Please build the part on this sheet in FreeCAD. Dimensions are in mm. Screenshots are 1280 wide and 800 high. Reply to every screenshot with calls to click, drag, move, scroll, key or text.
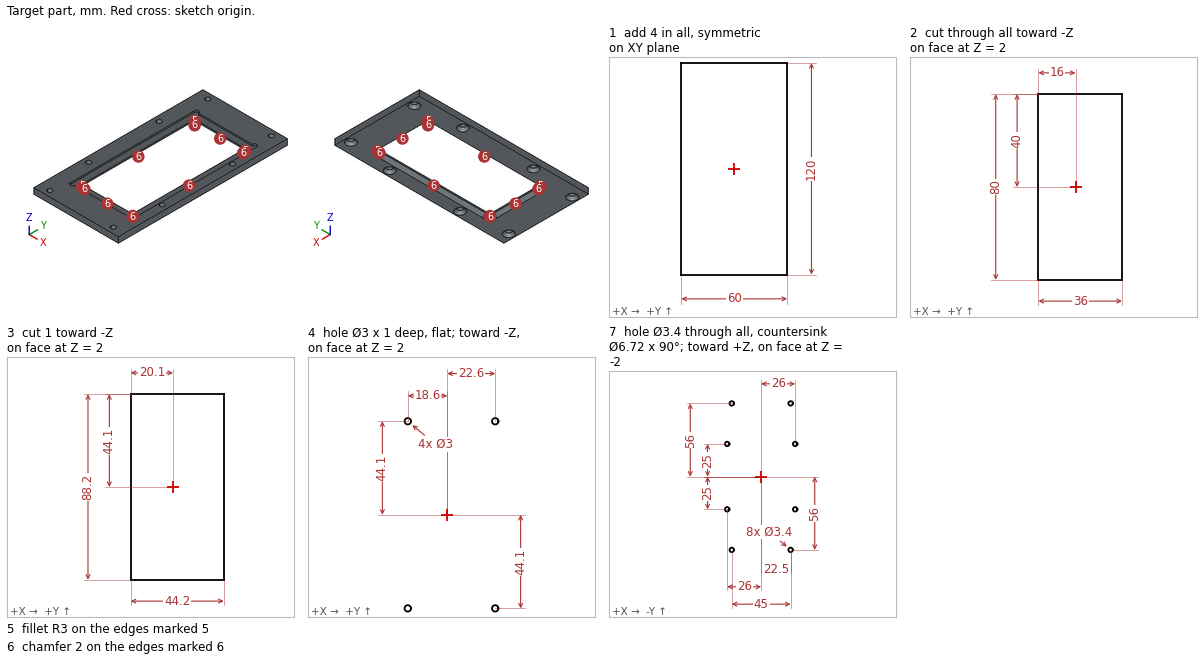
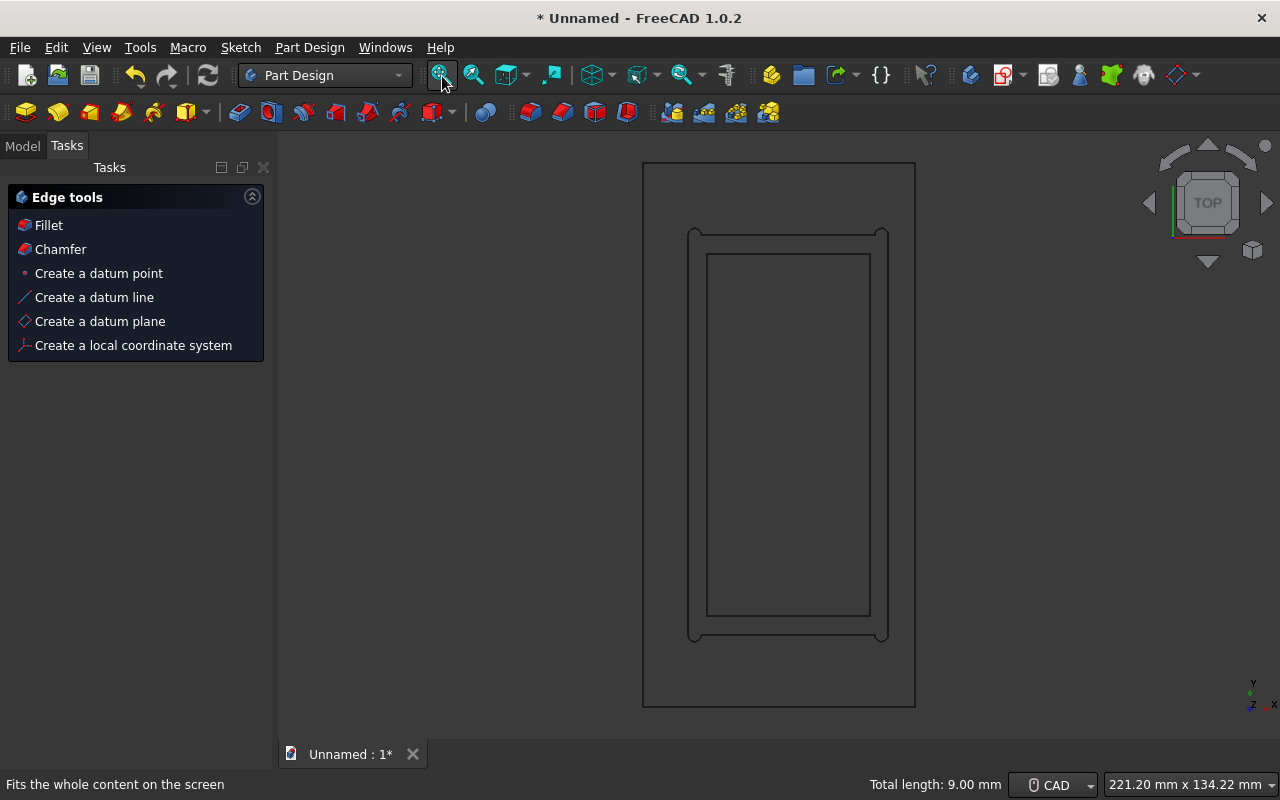
scroll(870, 253, up, 6)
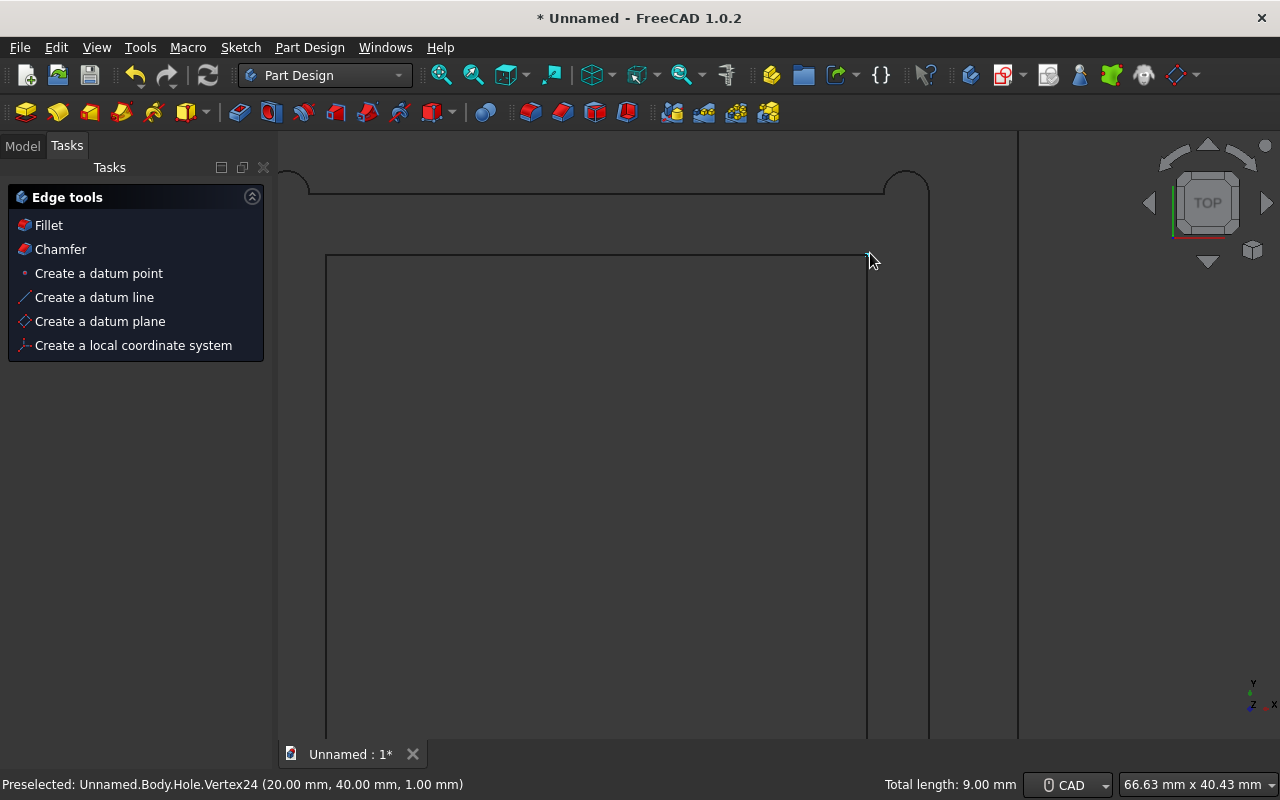
click(442, 76)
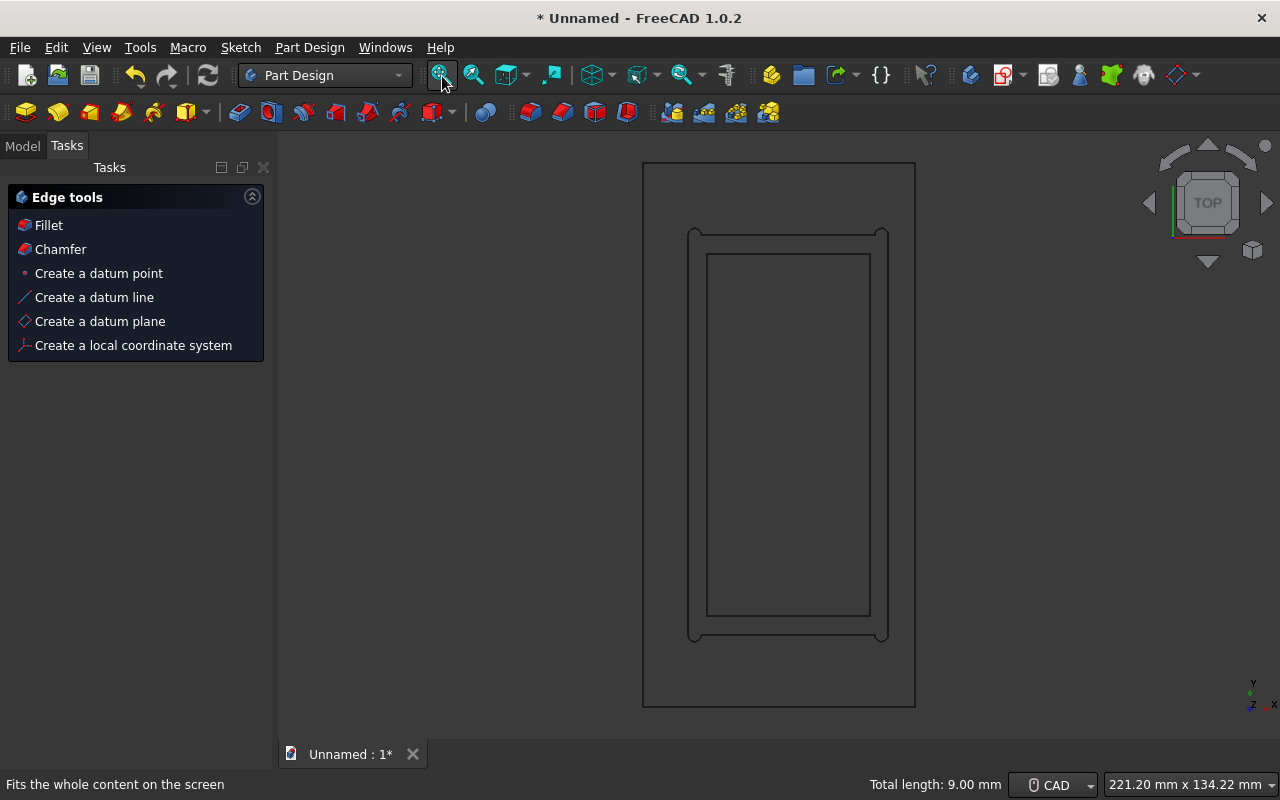
key(1)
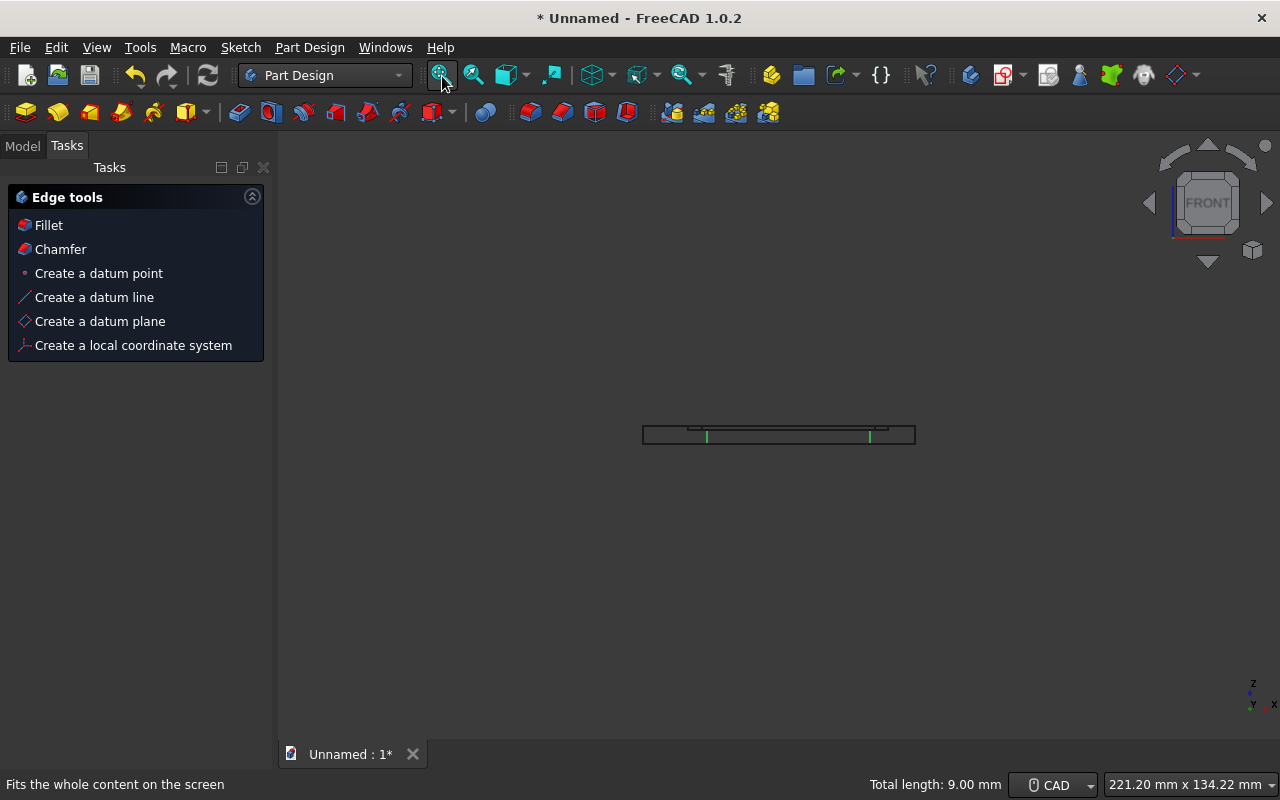
click(442, 76)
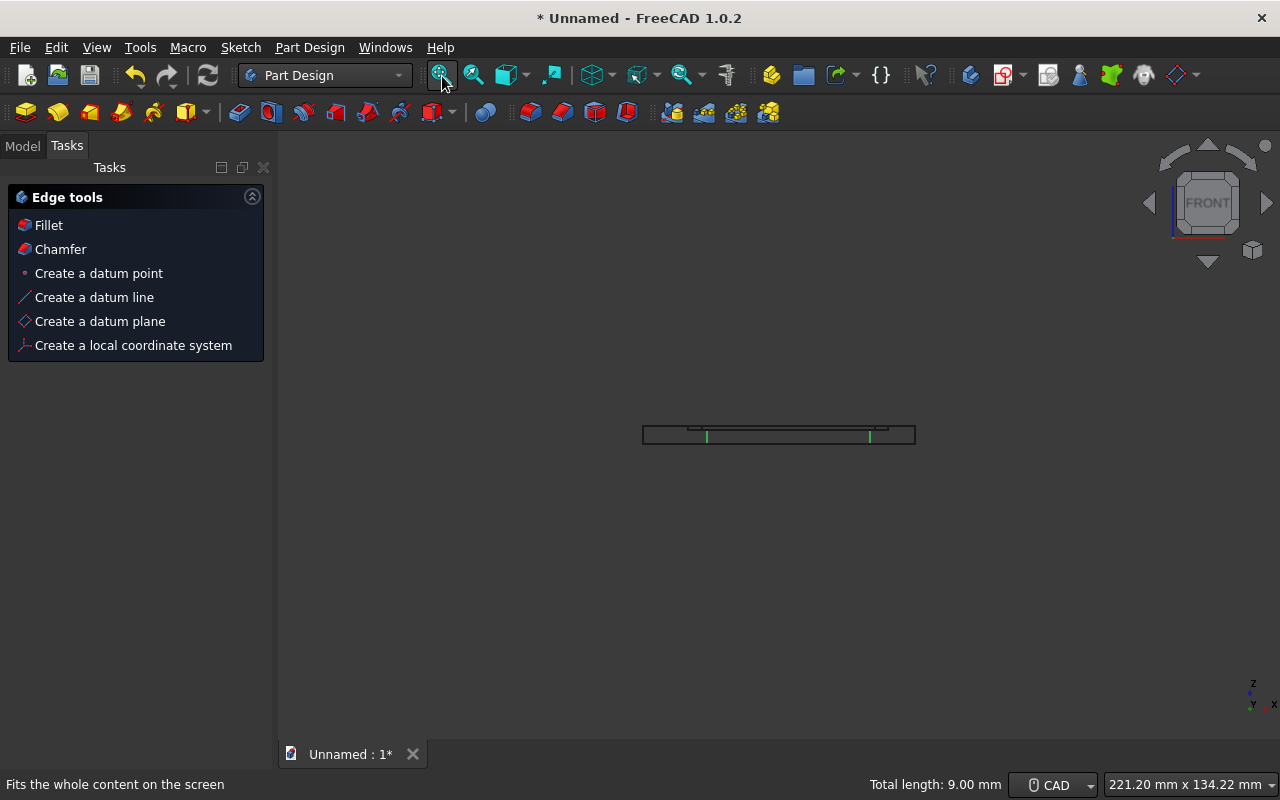
scroll(870, 436, up, 6)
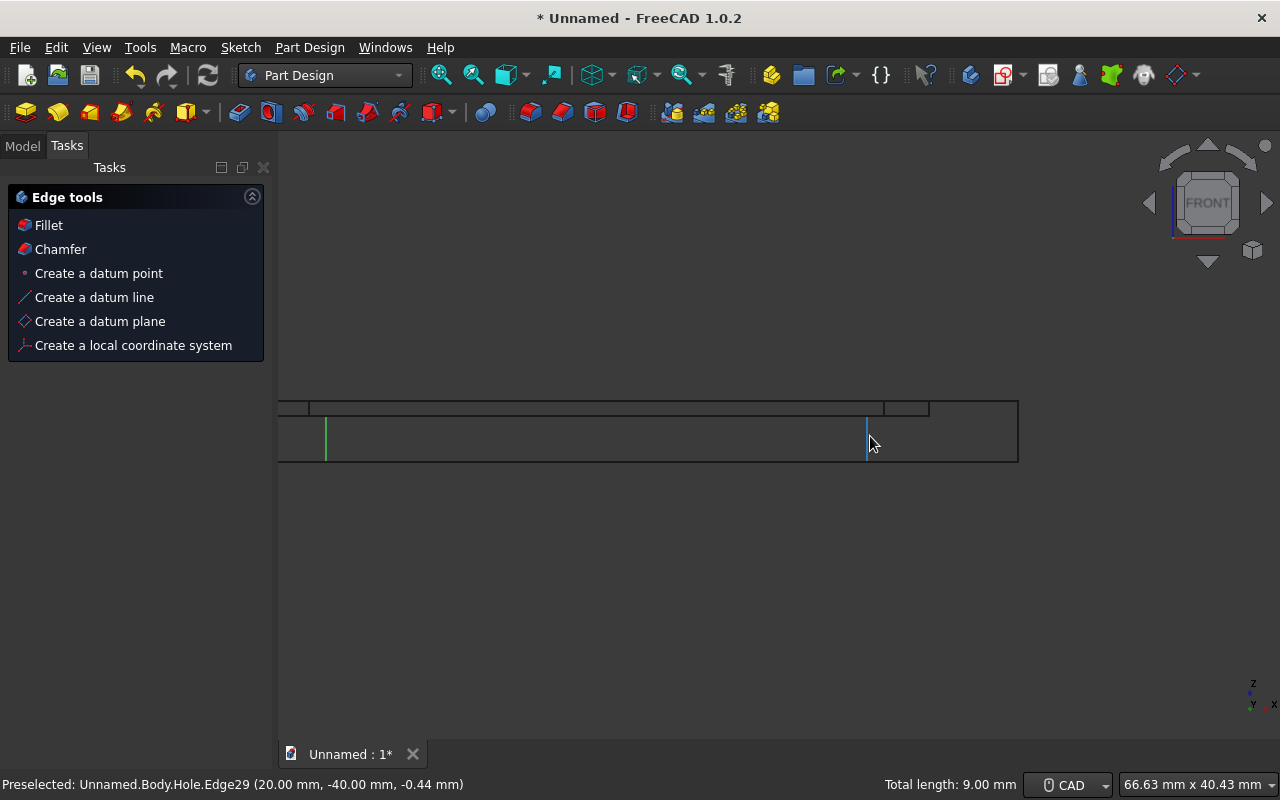
click(442, 76)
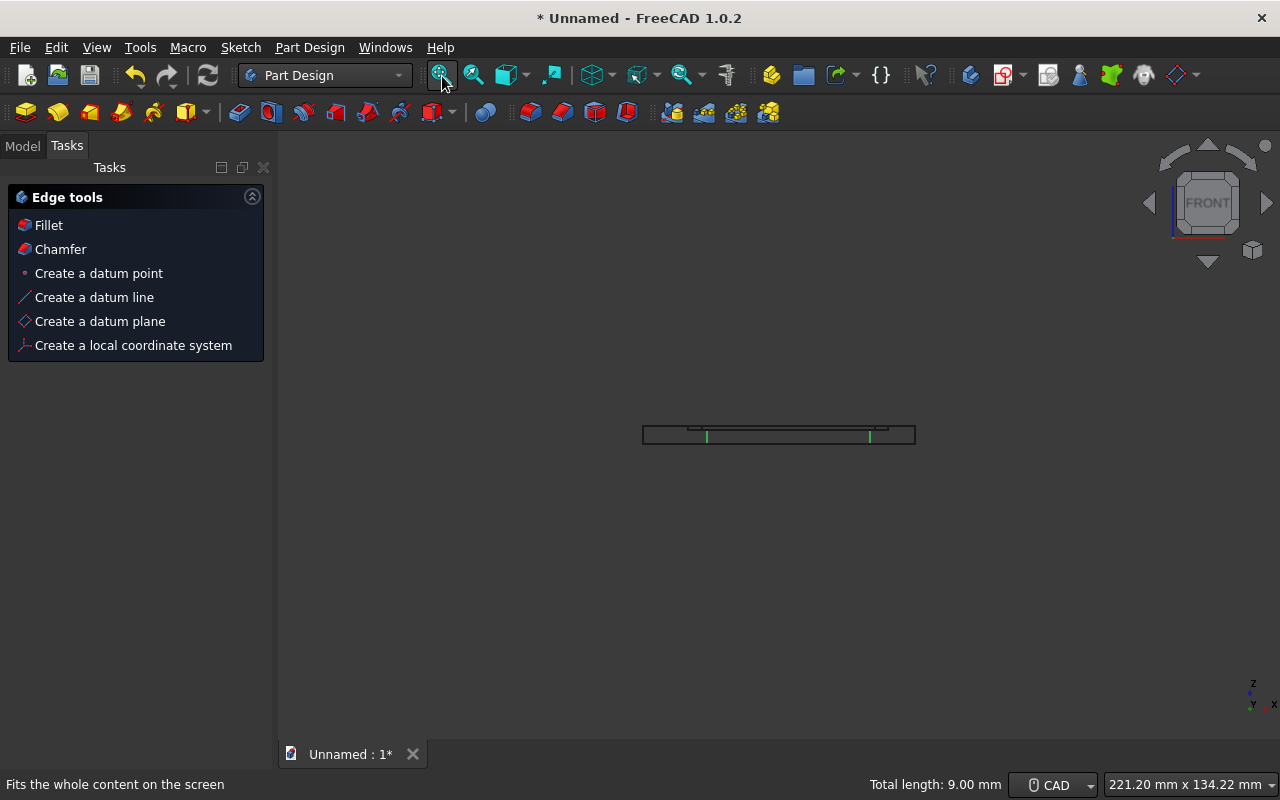
key(3)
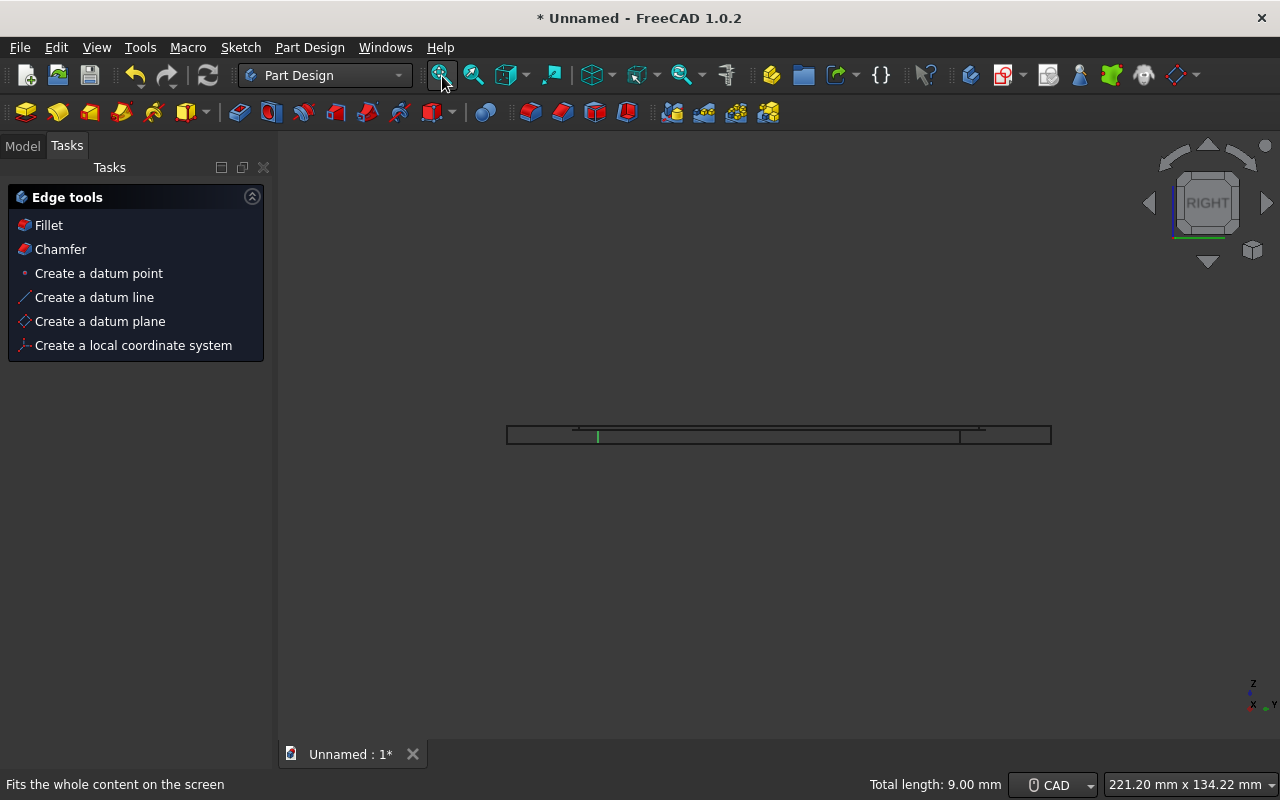
click(960, 436, ctrl)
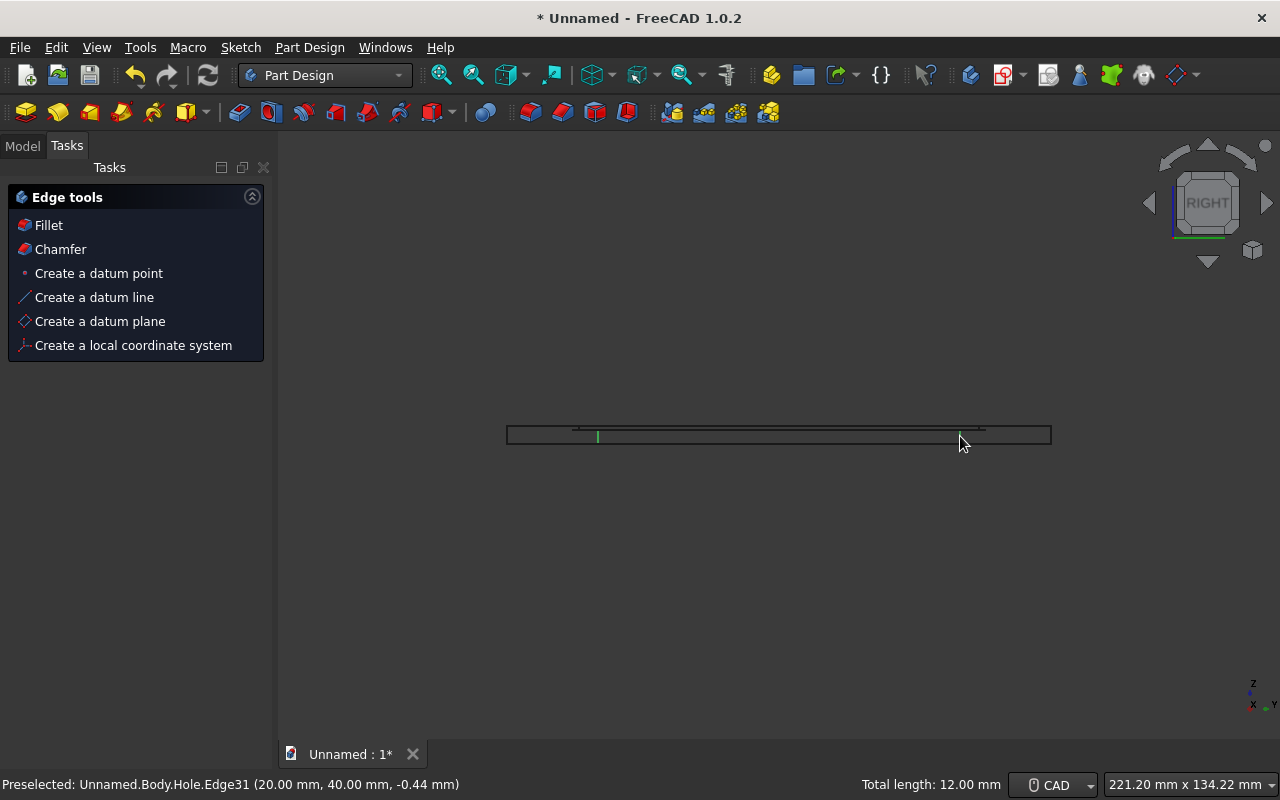
key(v)
key(1)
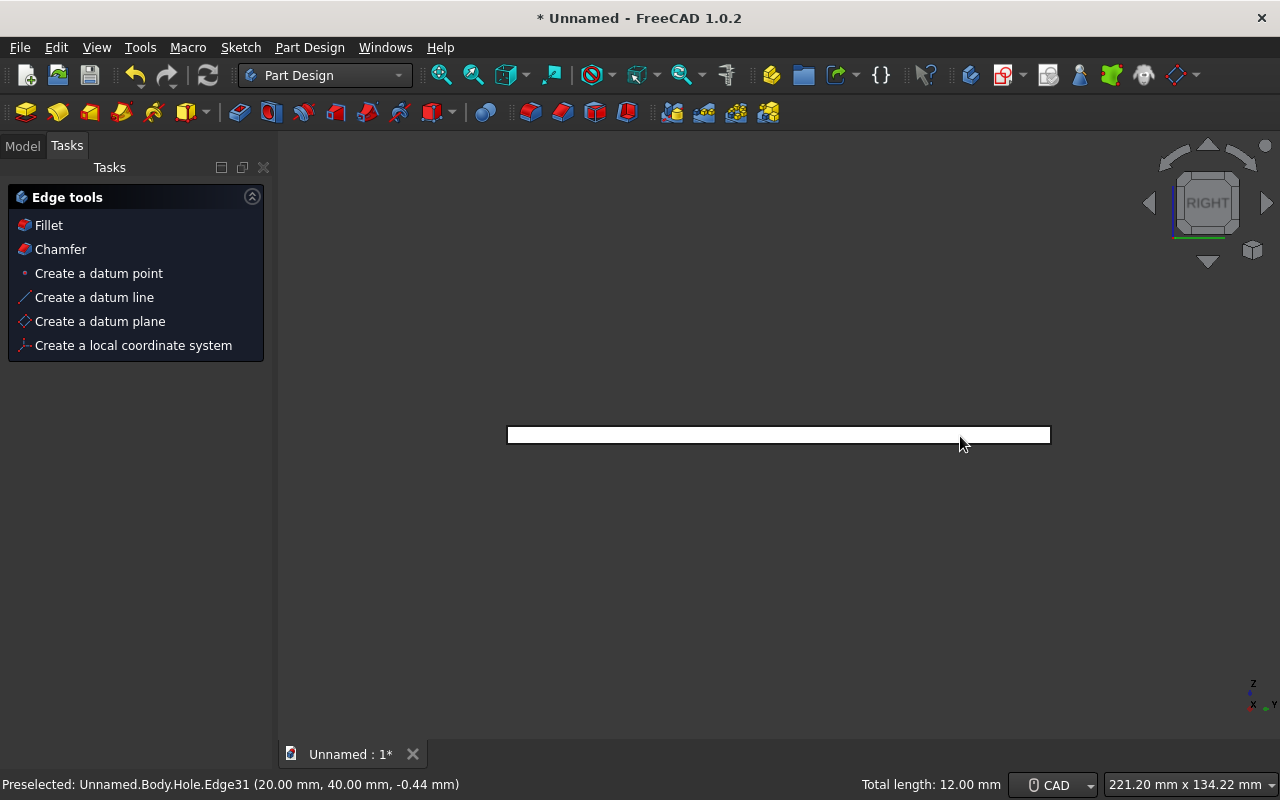
click(532, 112)